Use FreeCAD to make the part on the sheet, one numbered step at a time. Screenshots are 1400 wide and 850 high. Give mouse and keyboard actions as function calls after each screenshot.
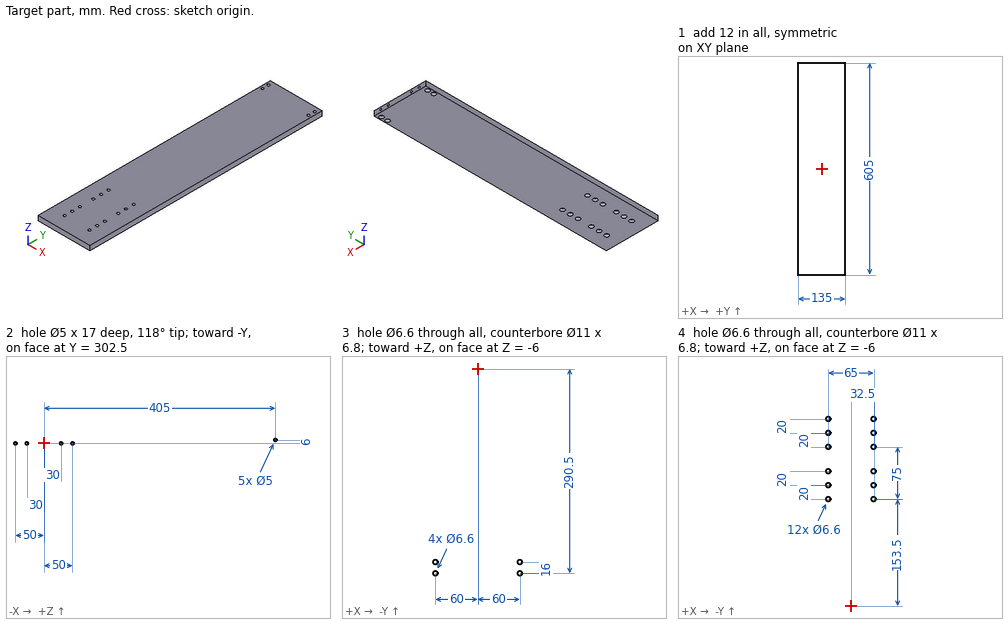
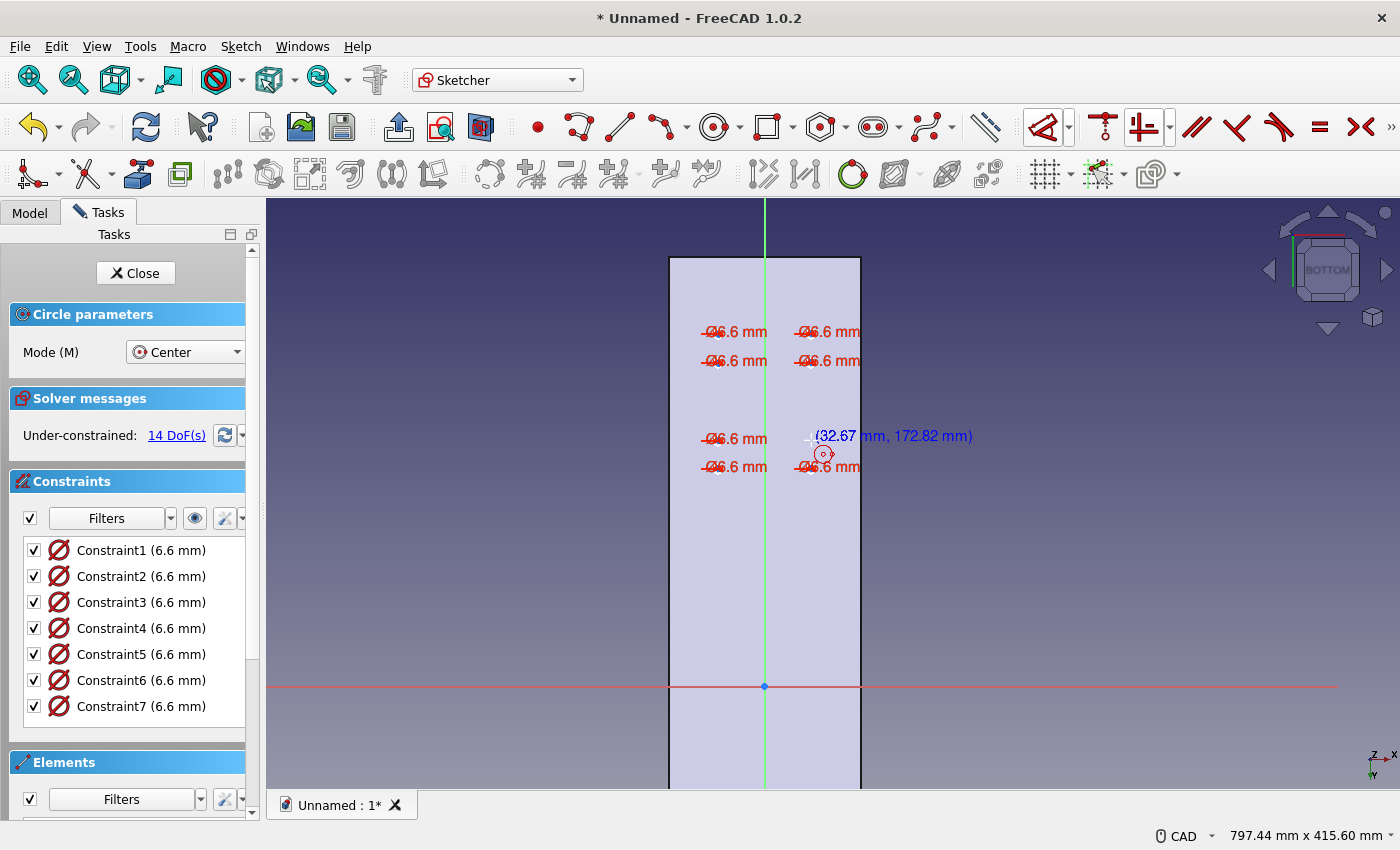
click(811, 440)
move(814, 437)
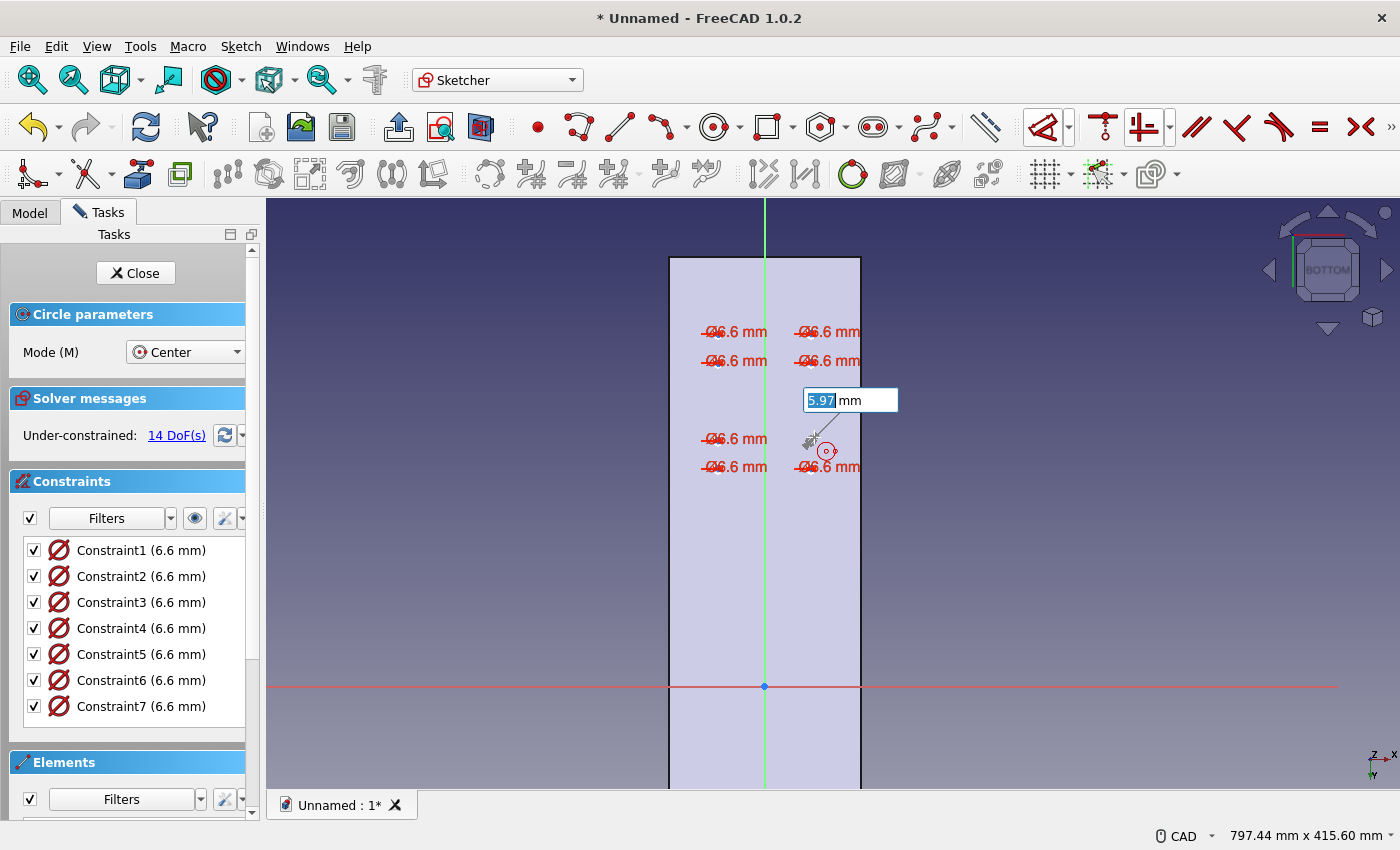
text(6.6)
key(Return)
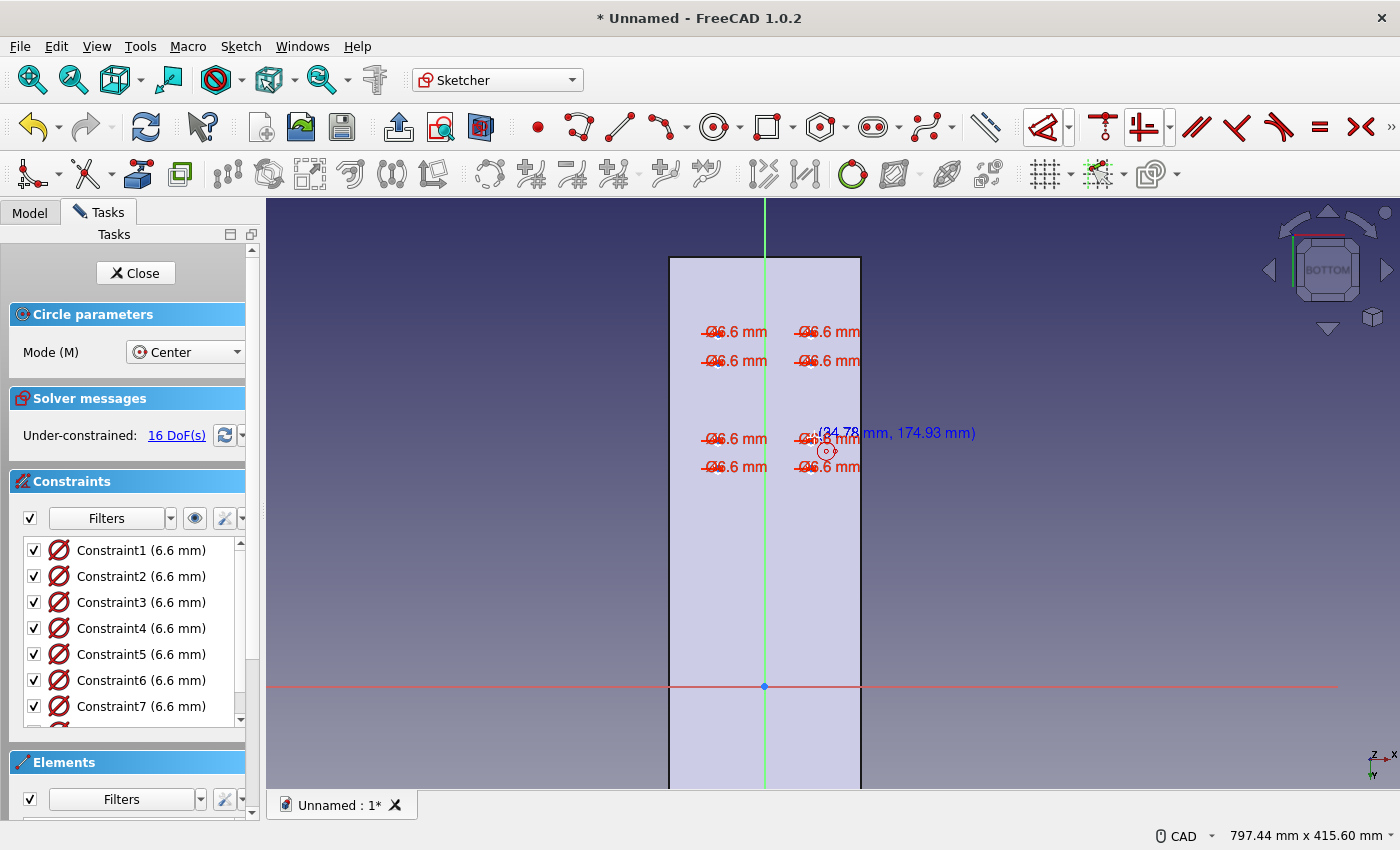
scroll(718, 305, up, 8)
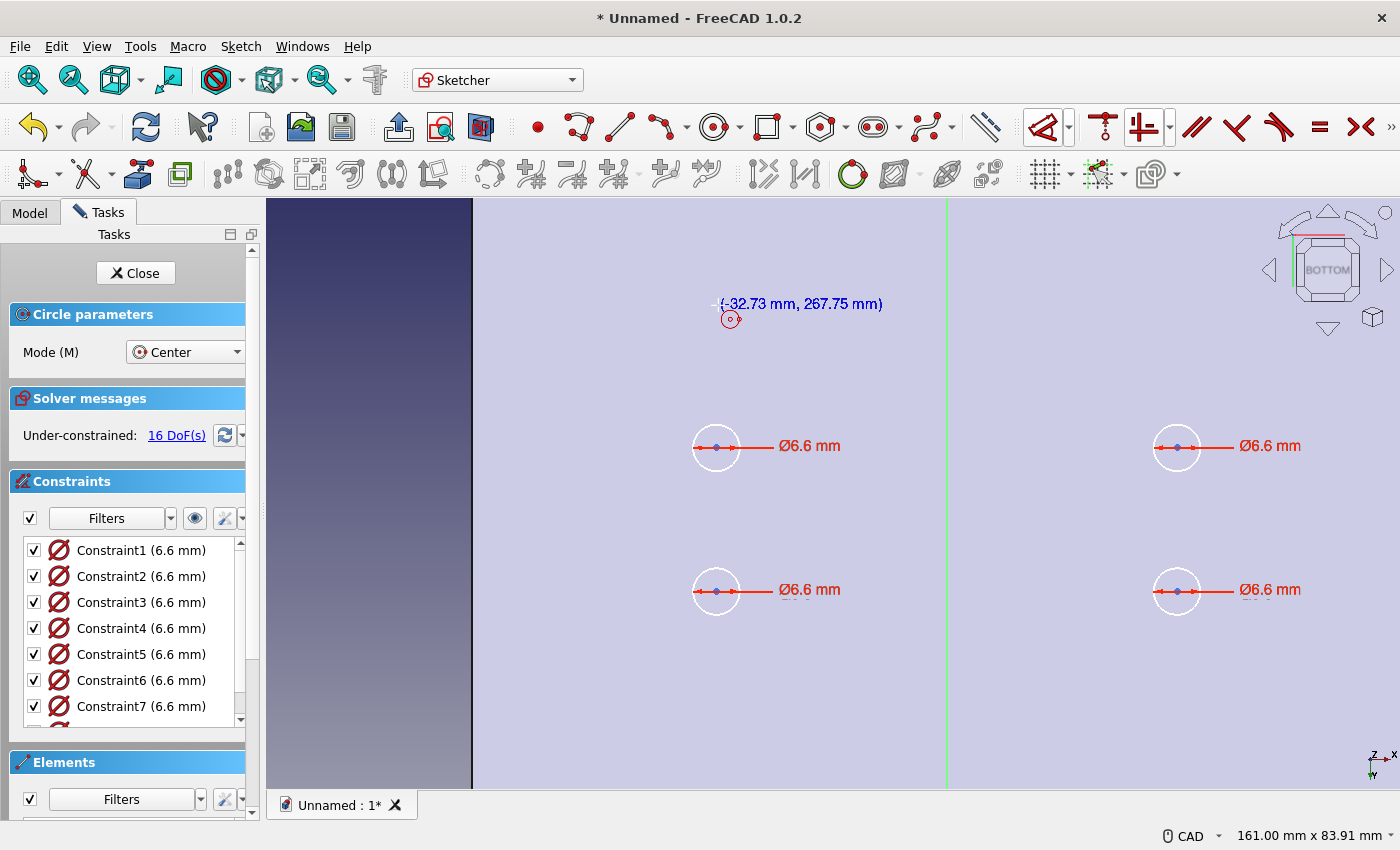
scroll(718, 305, down, 8)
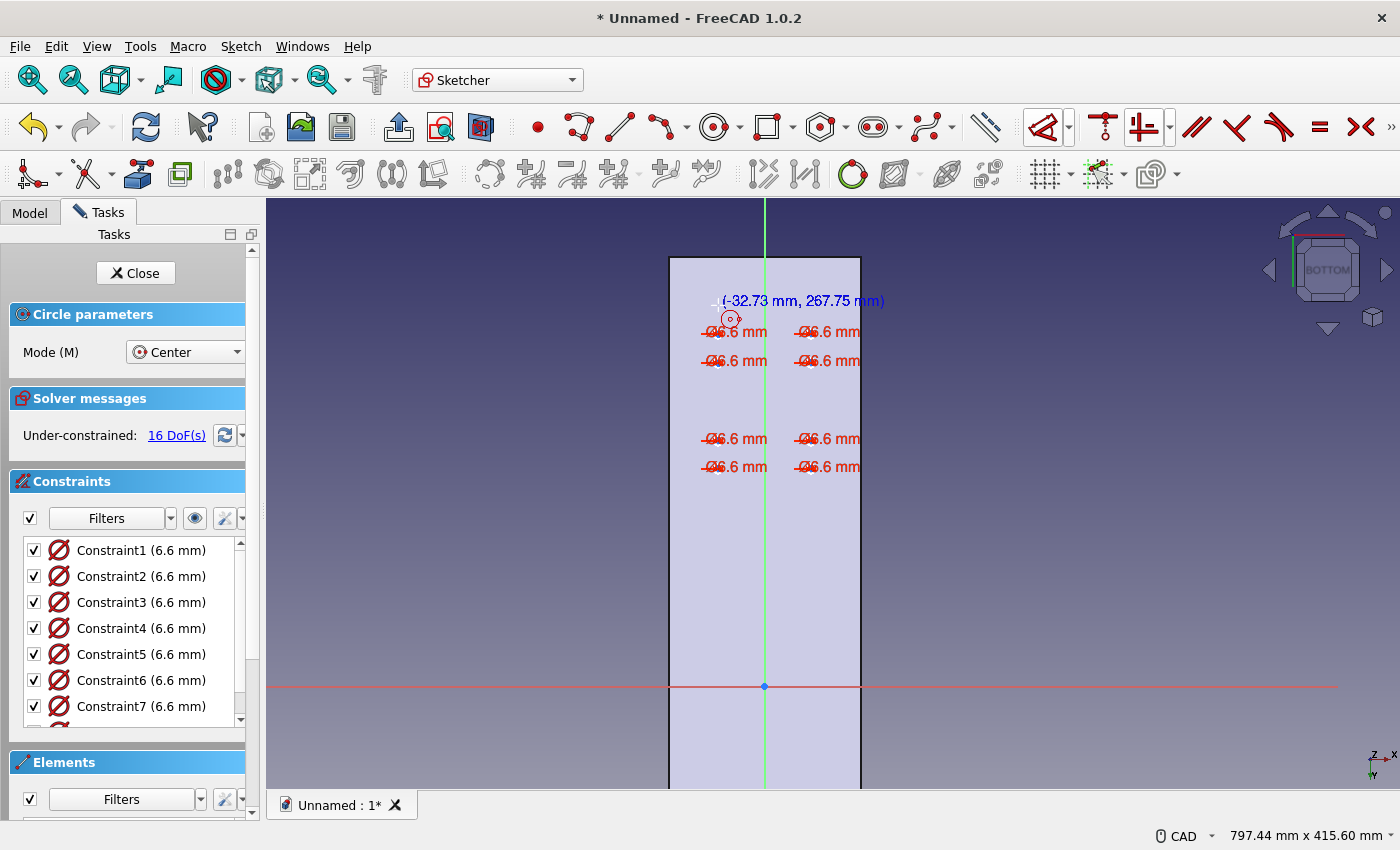
click(718, 305)
move(722, 302)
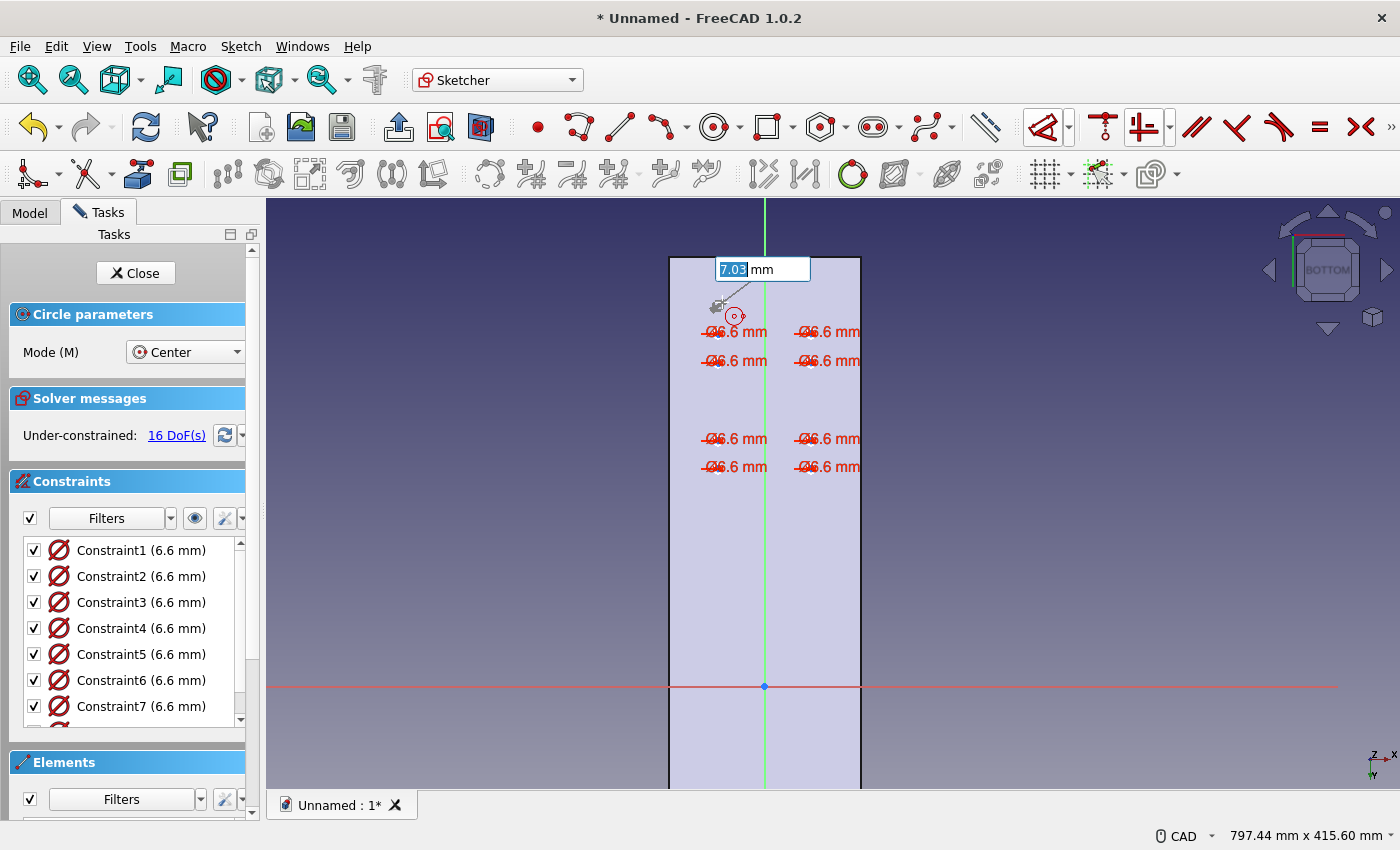
text(6.6)
key(Return)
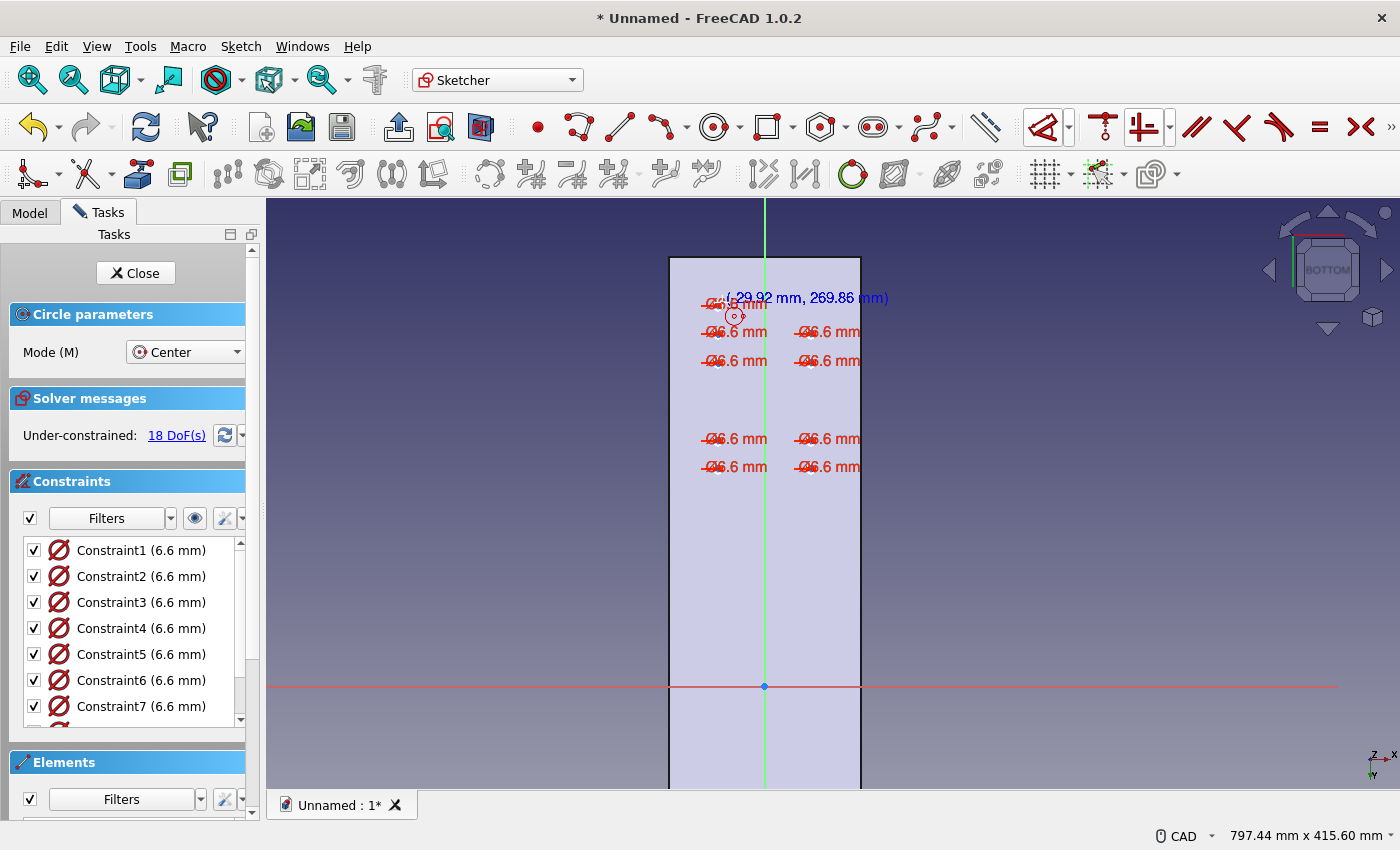
scroll(718, 412, up, 8)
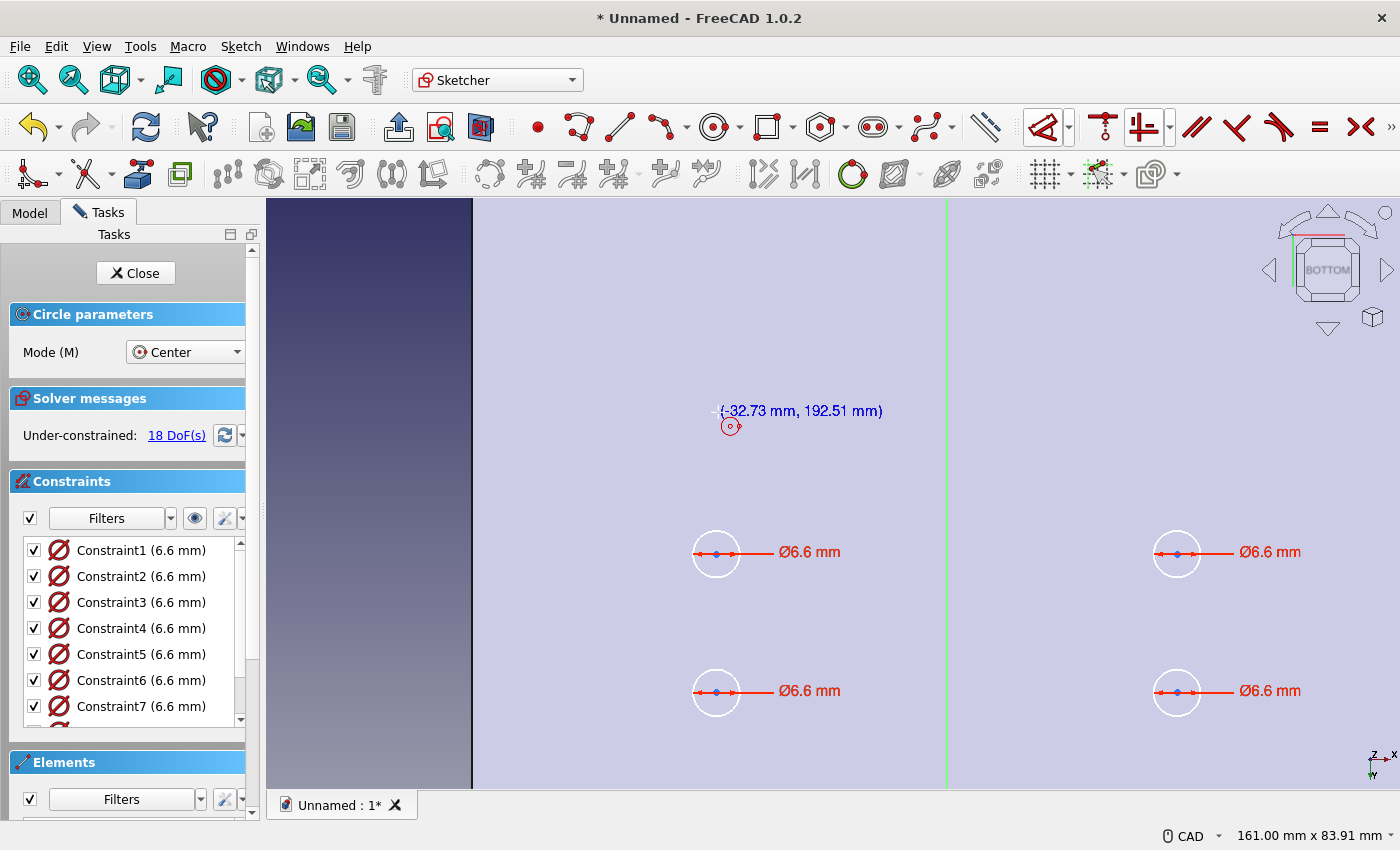
scroll(718, 412, down, 8)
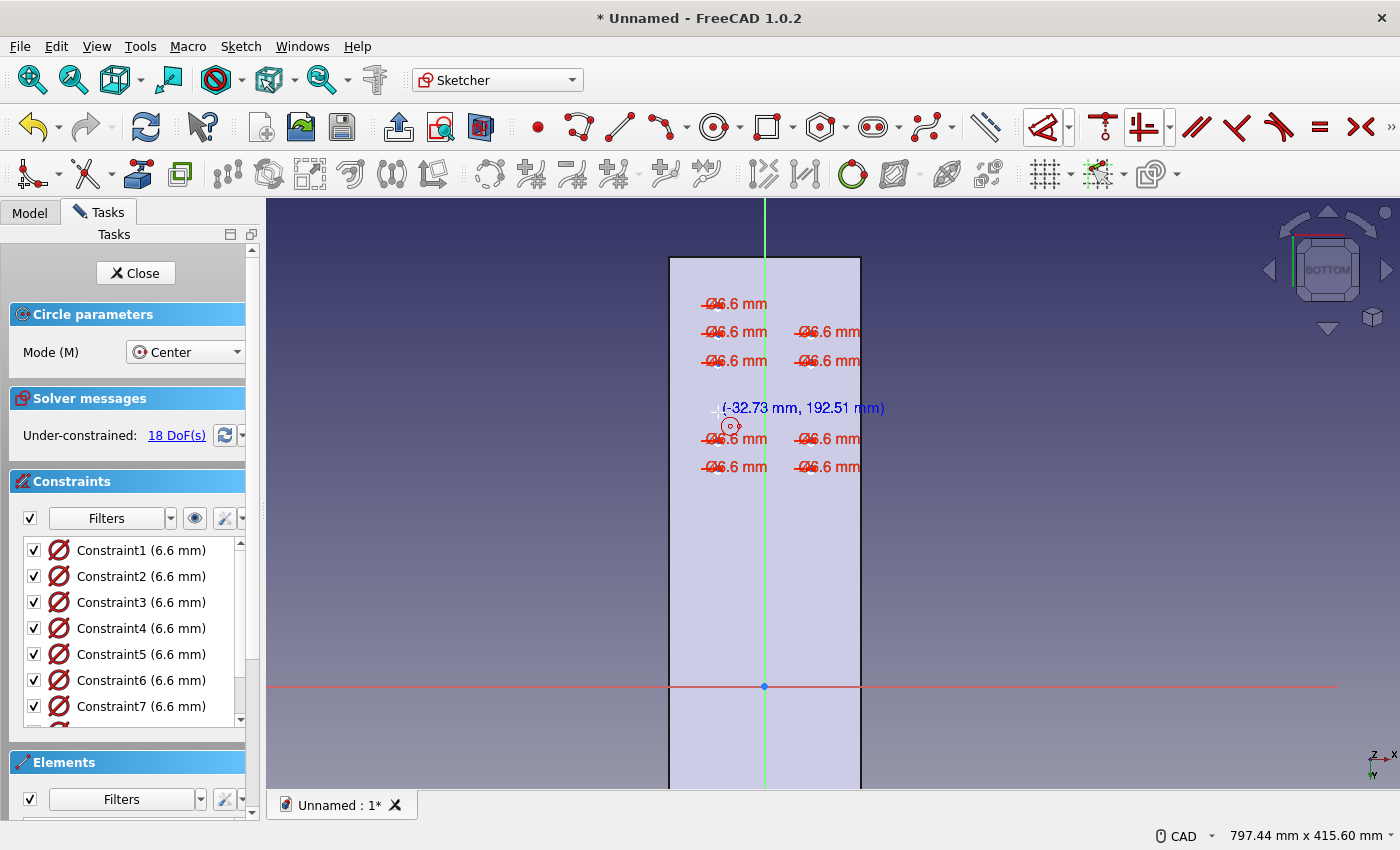
click(718, 412)
move(722, 408)